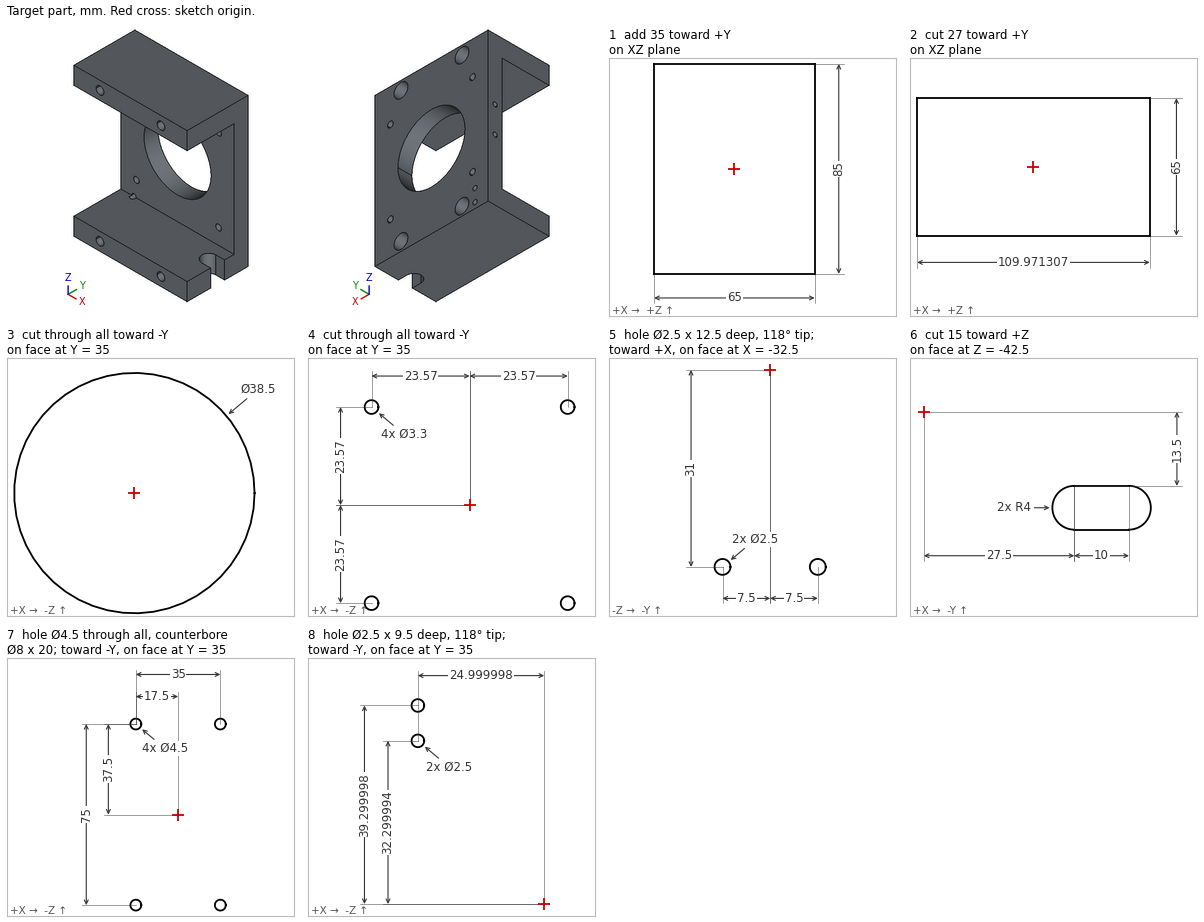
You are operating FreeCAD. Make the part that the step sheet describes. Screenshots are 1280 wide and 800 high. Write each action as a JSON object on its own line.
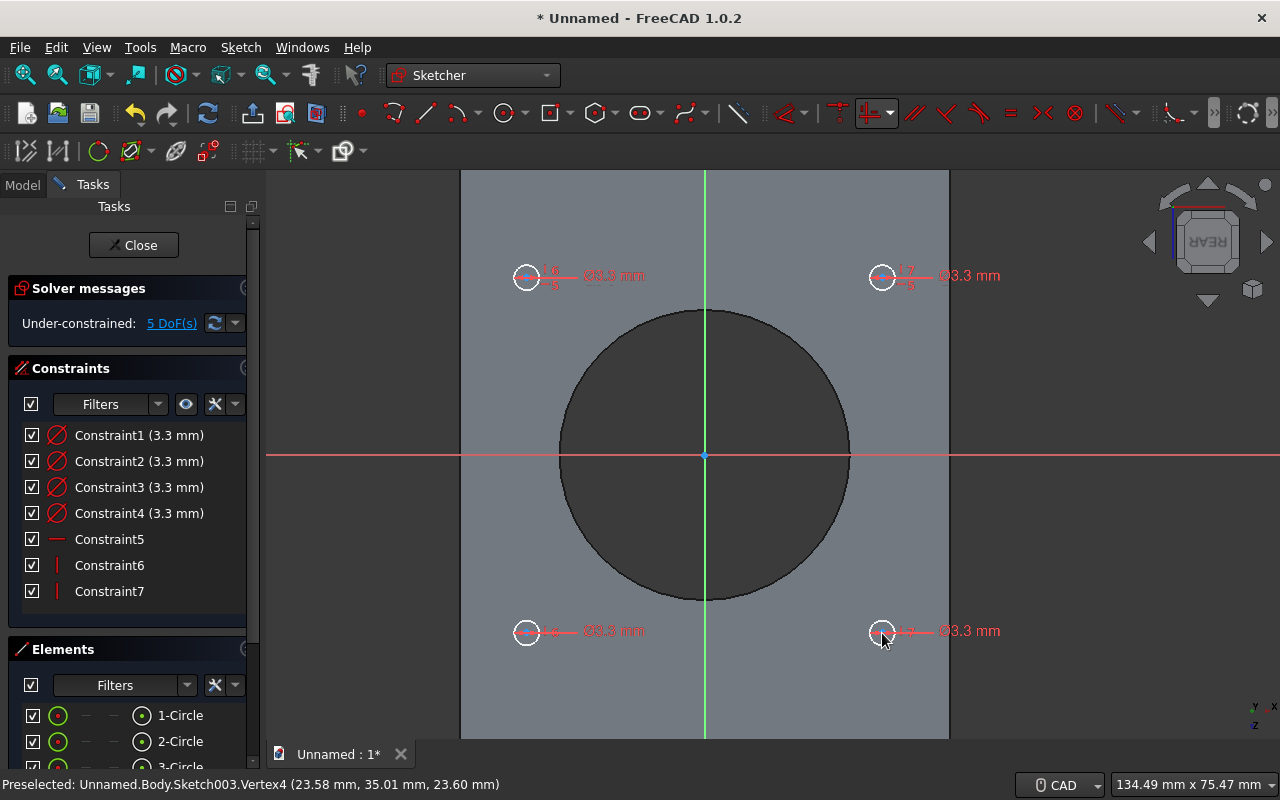
{"action": "left_click", "coordinate": [527, 633]}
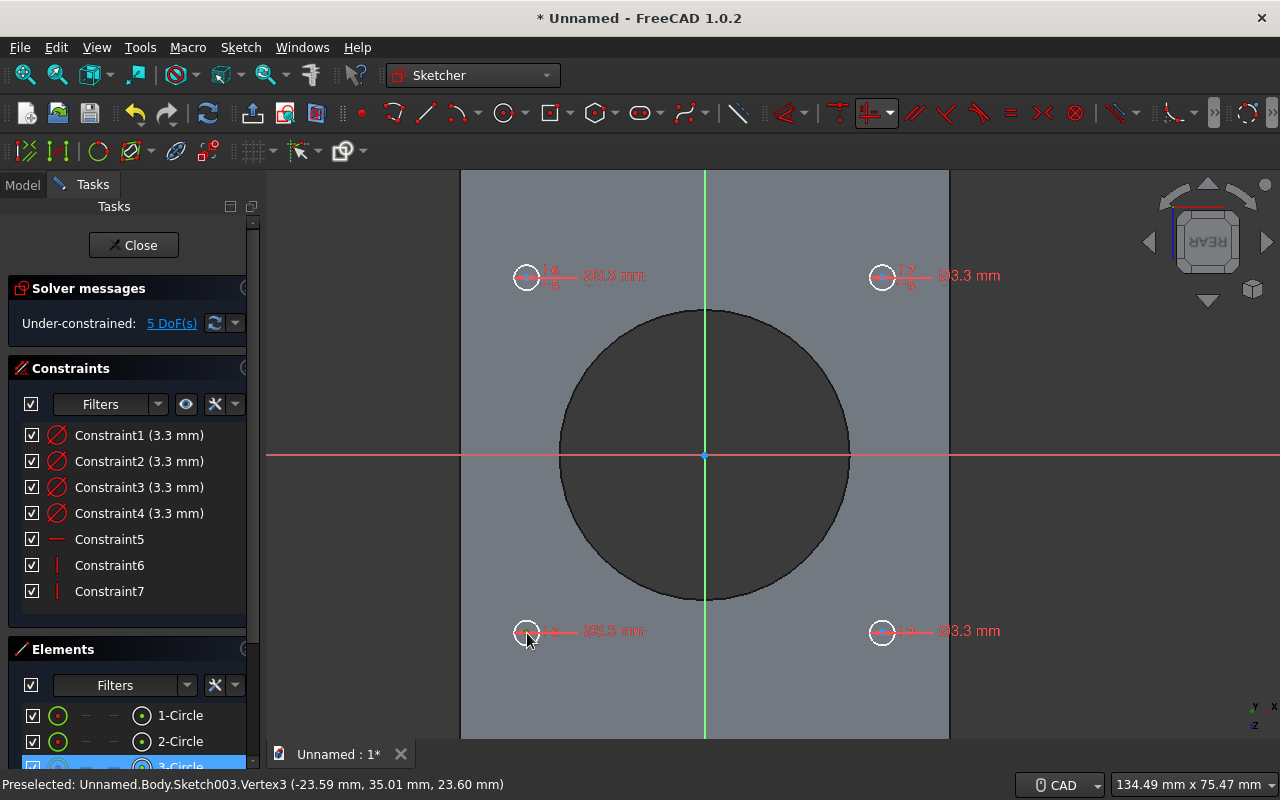
{"action": "left_click", "coordinate": [882, 633]}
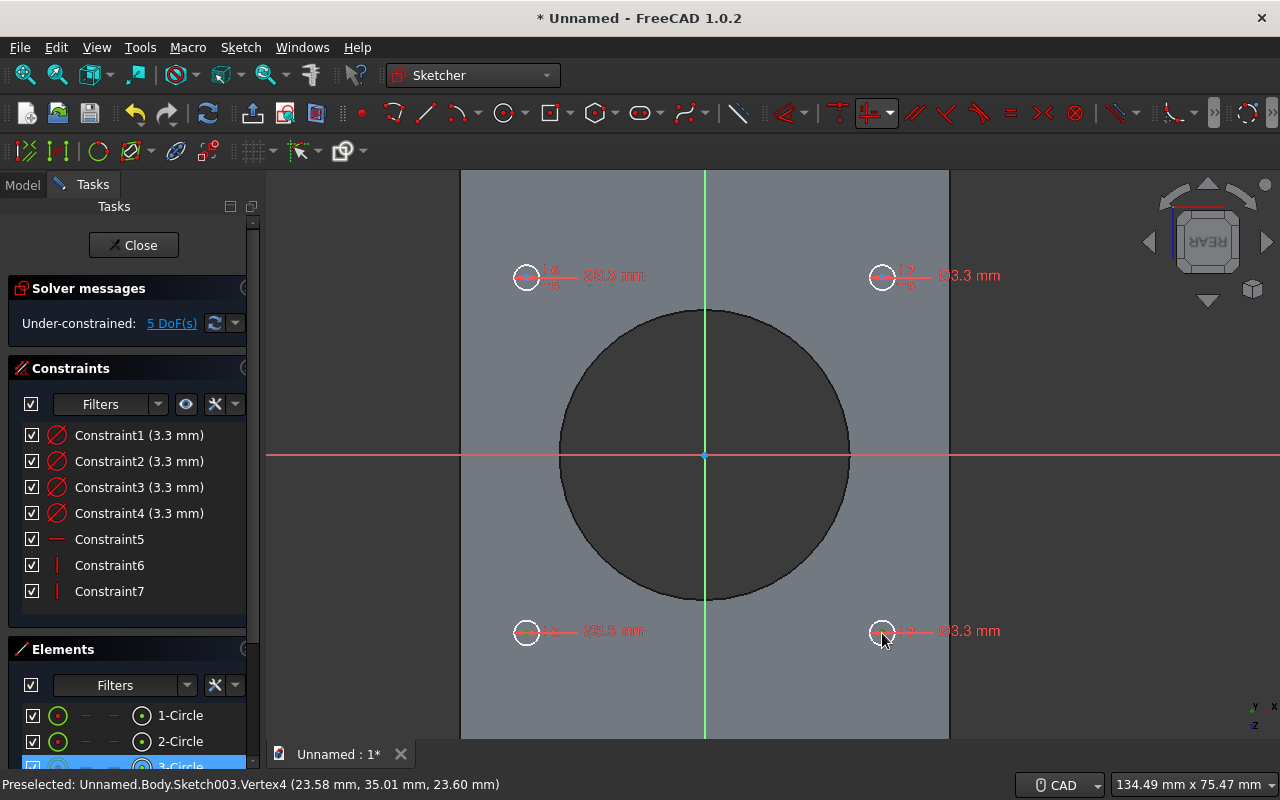
{"action": "key", "text": "h"}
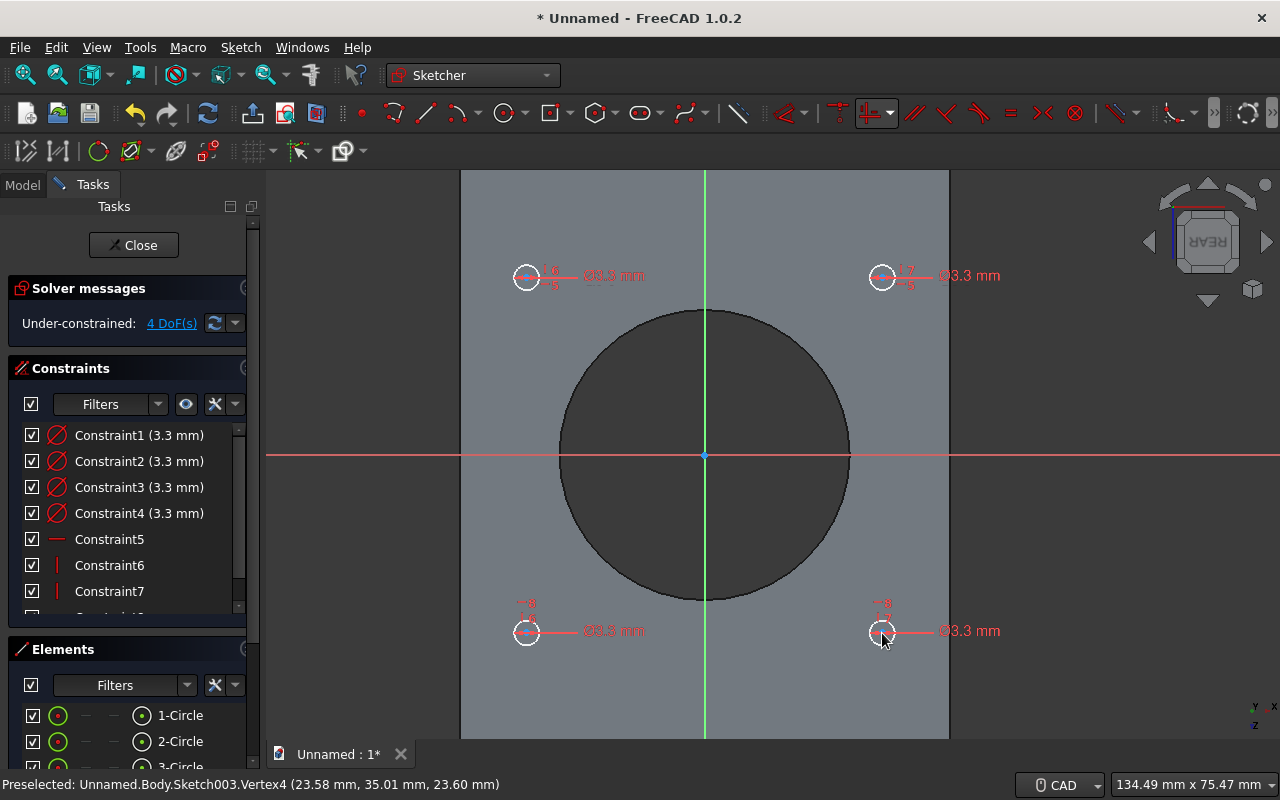
{"action": "left_click", "coordinate": [784, 114]}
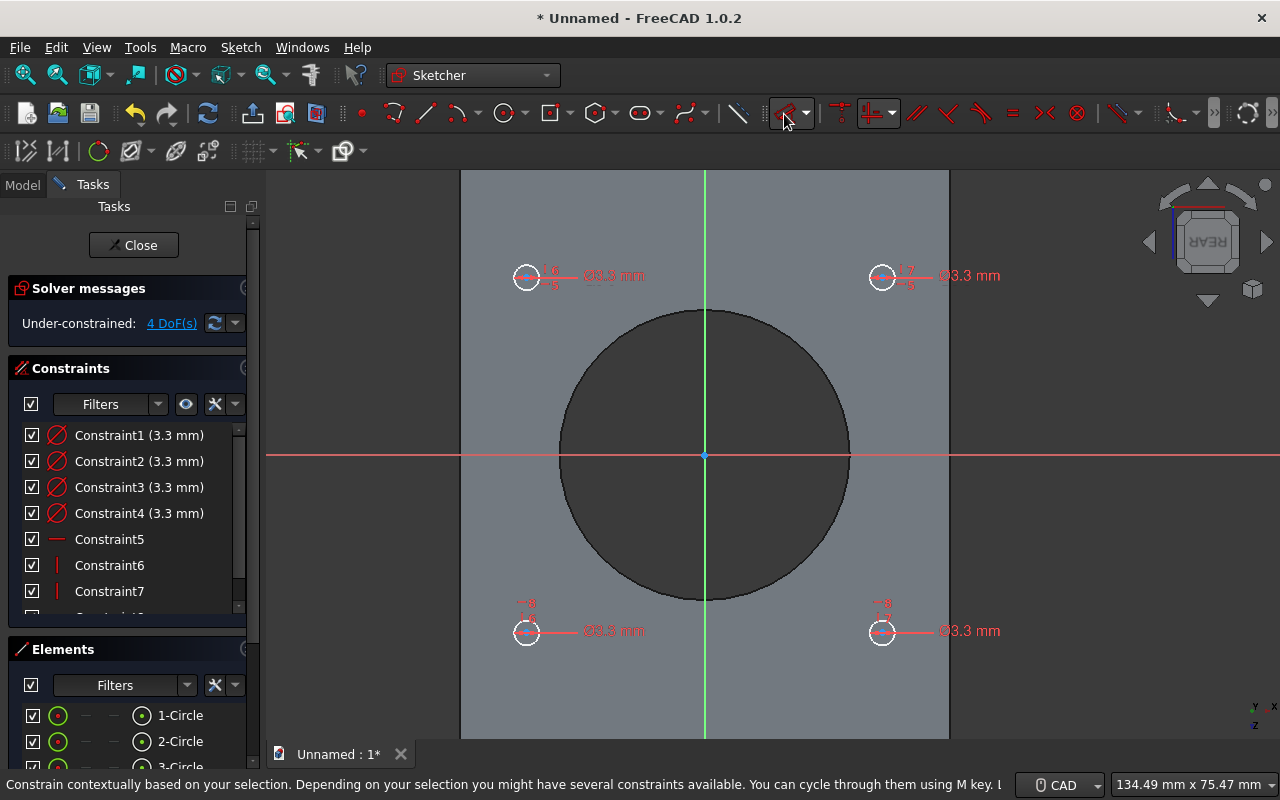
{"action": "left_click", "coordinate": [527, 278]}
{"action": "left_click", "coordinate": [616, 244]}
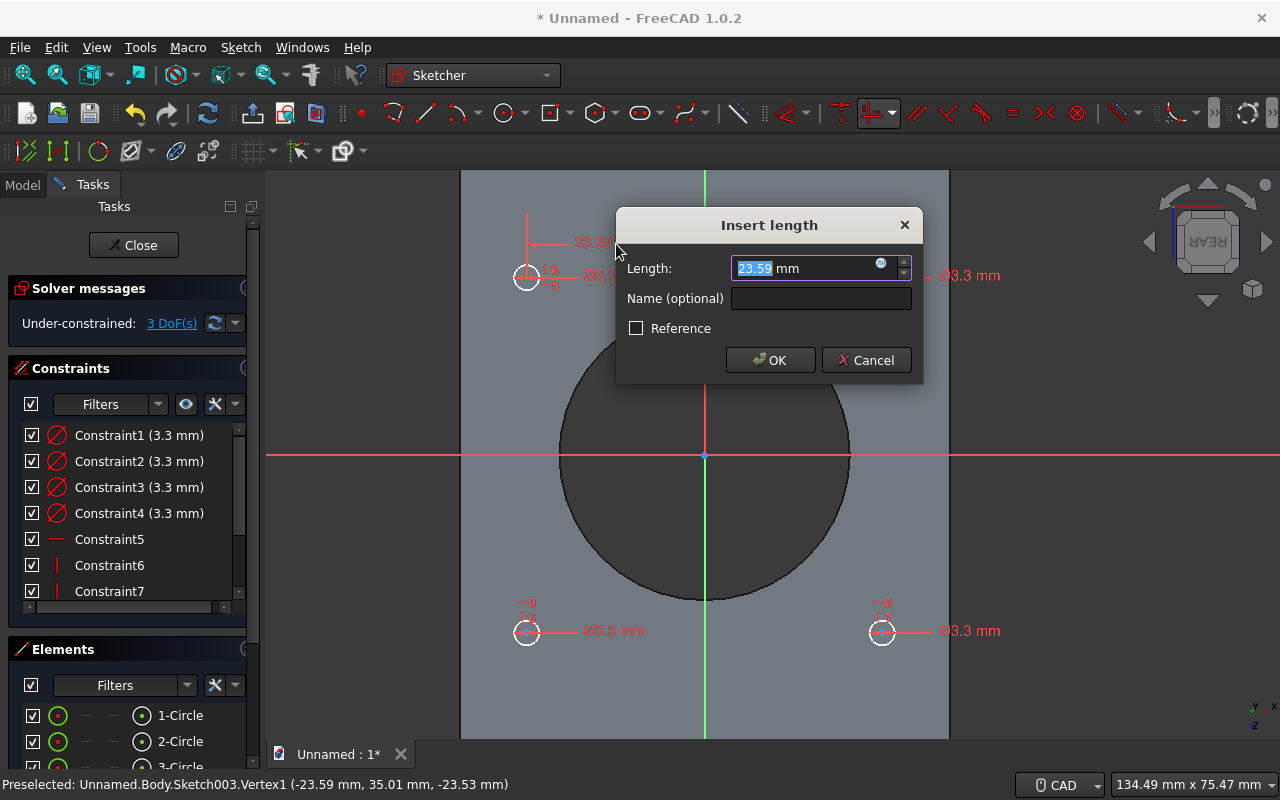
{"action": "type", "text": "23.57"}
{"action": "key", "text": "Return"}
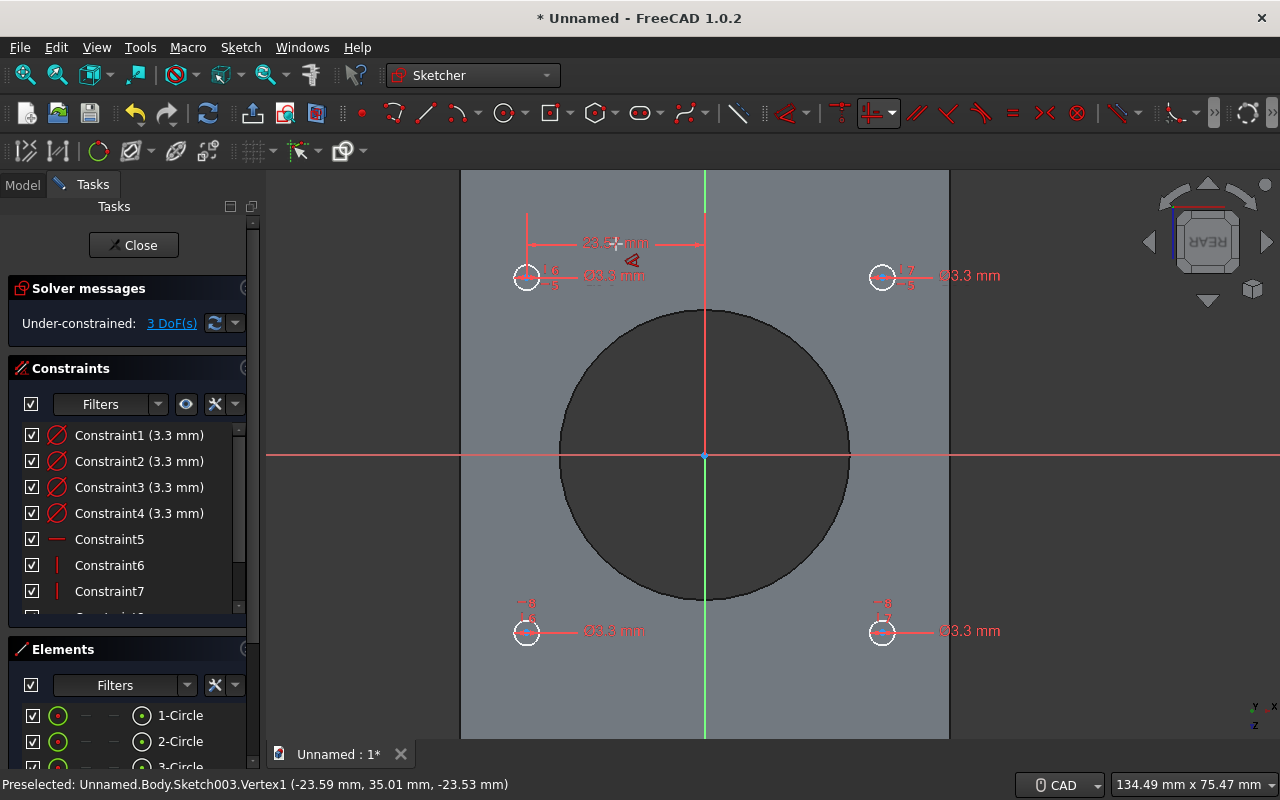
{"action": "left_click", "coordinate": [527, 278]}
{"action": "left_click", "coordinate": [493, 366]}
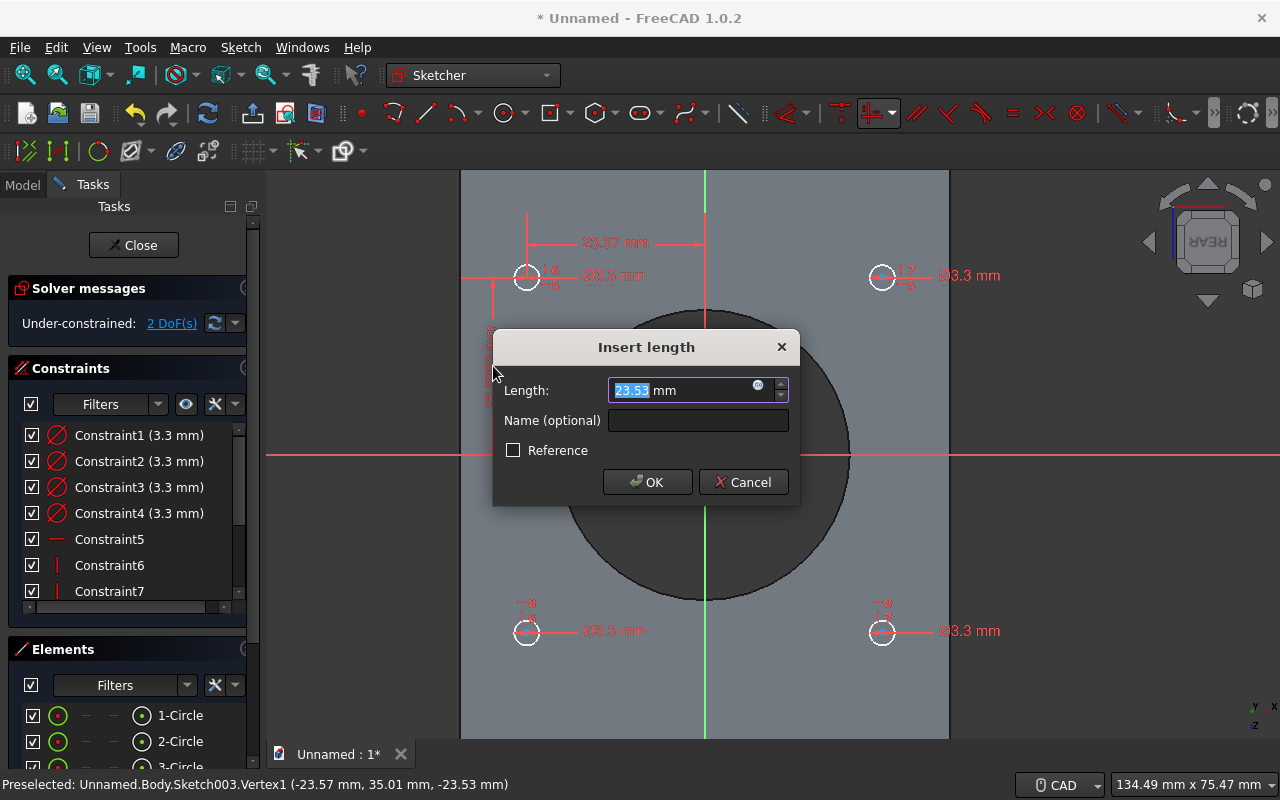
{"action": "type", "text": "23.57"}
{"action": "key", "text": "Return"}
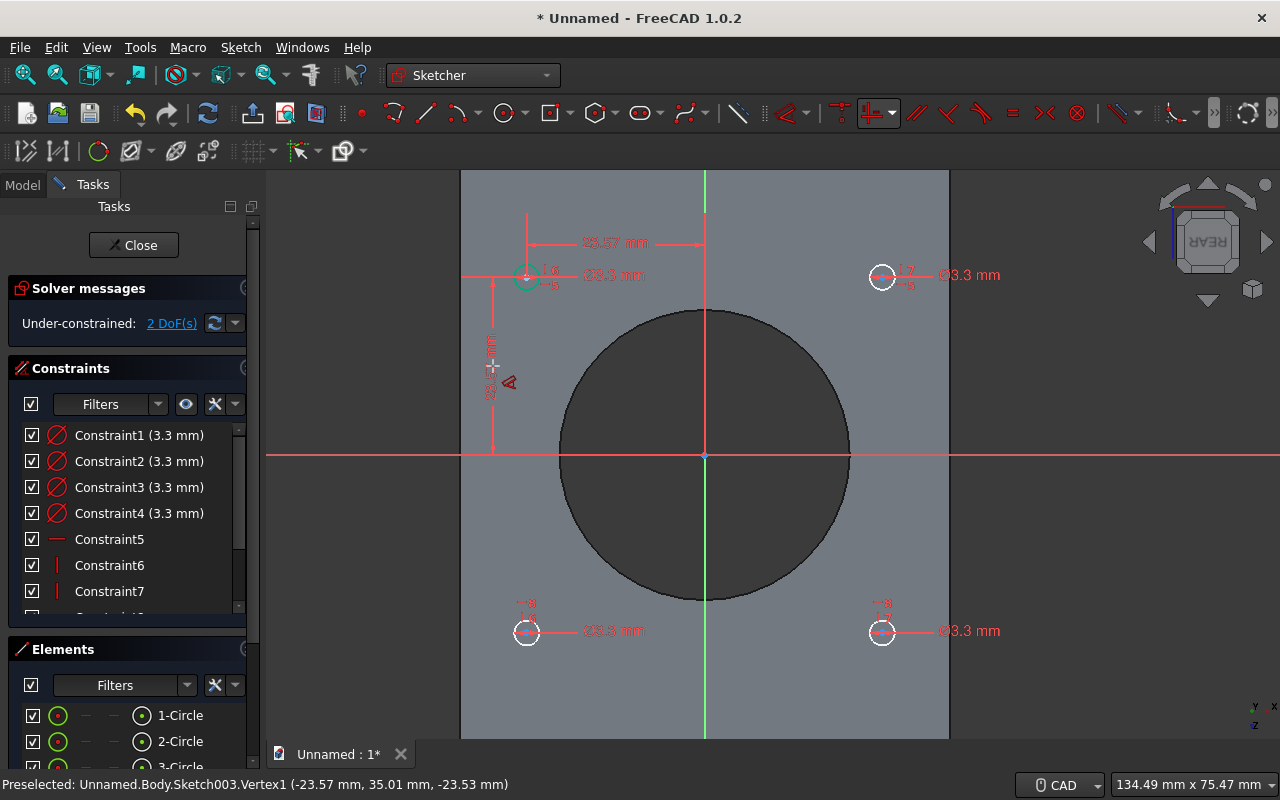
{"action": "left_click", "coordinate": [882, 277]}
{"action": "left_click", "coordinate": [793, 243]}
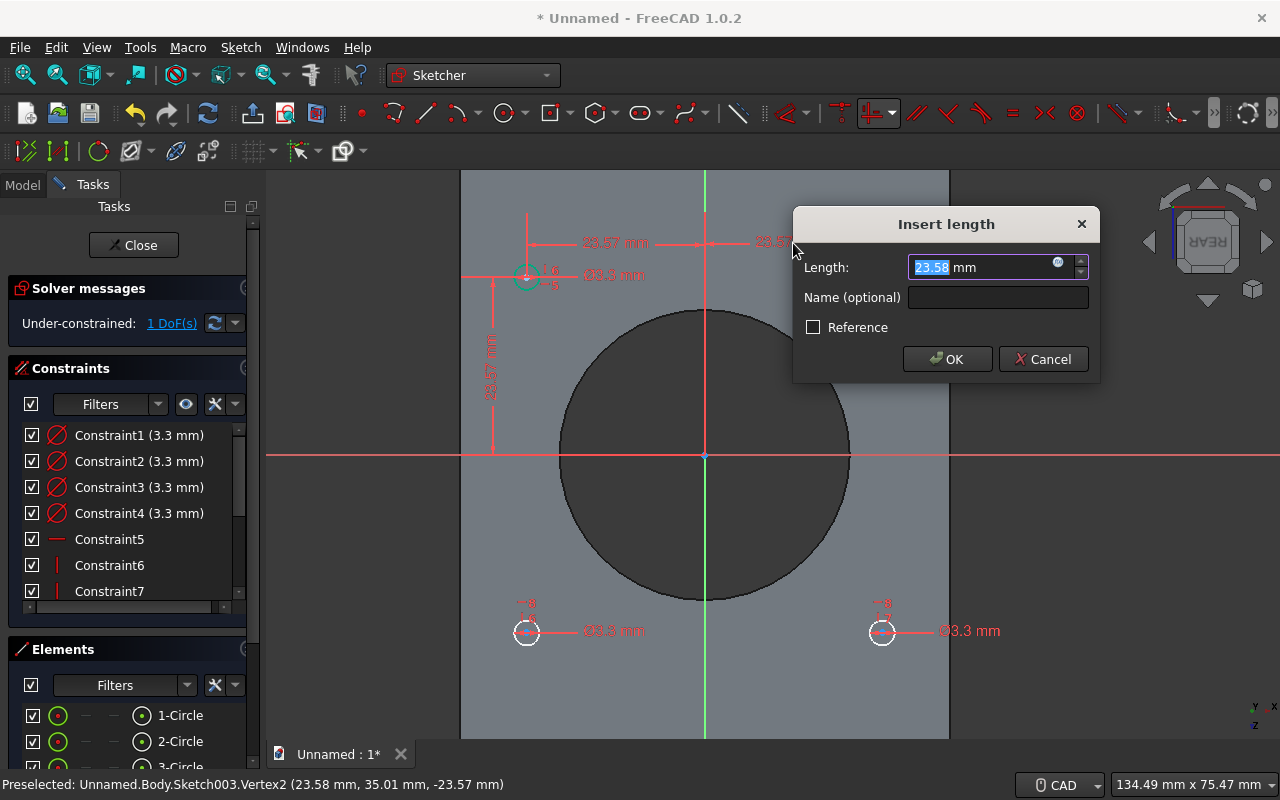
{"action": "type", "text": "23.57"}
{"action": "key", "text": "Return"}